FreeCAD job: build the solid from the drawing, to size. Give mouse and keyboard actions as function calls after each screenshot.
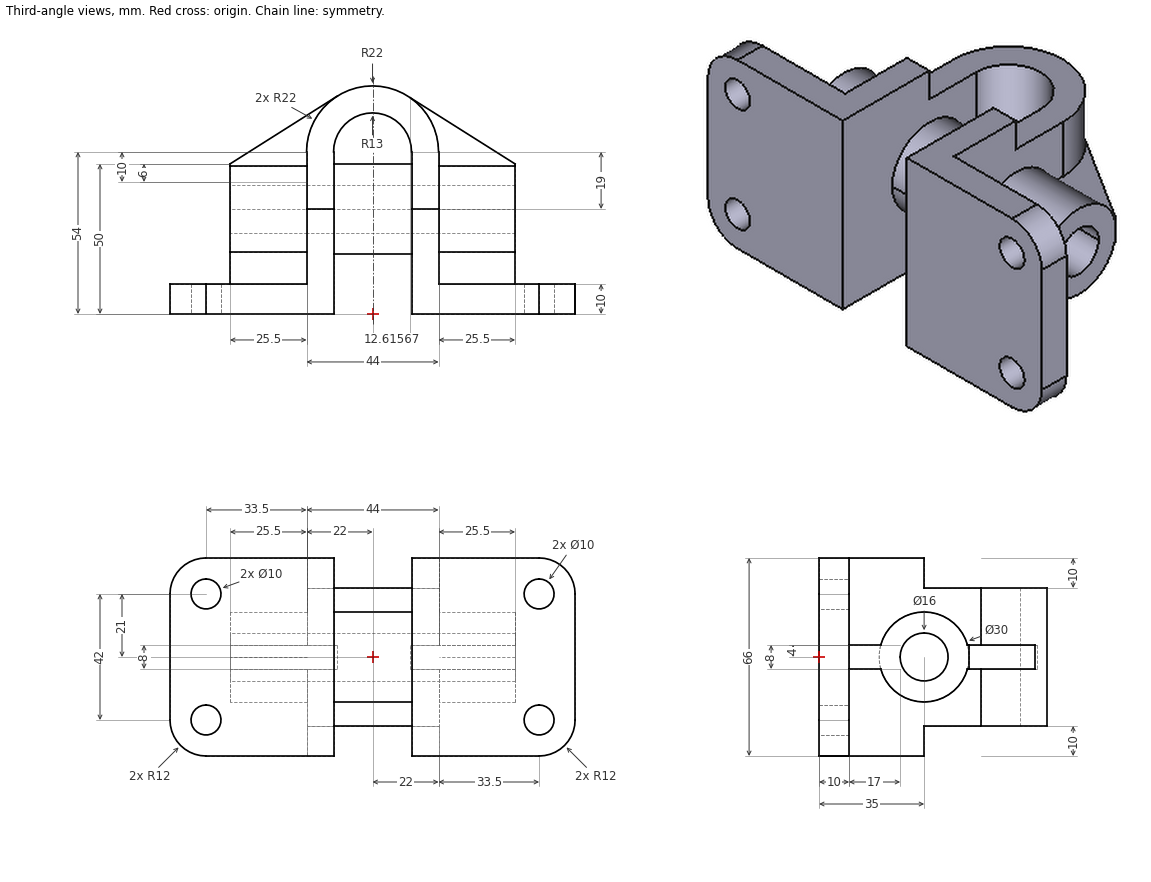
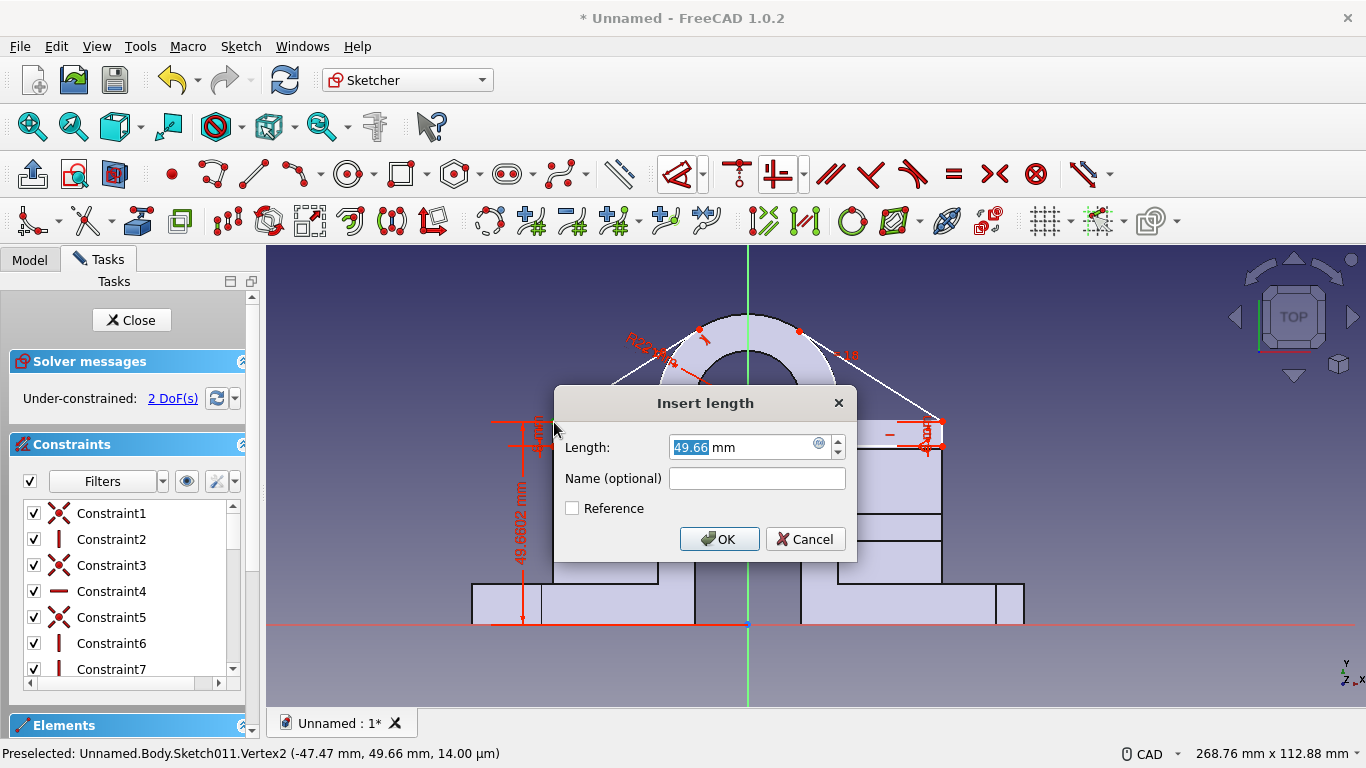
text(50)
key(Return)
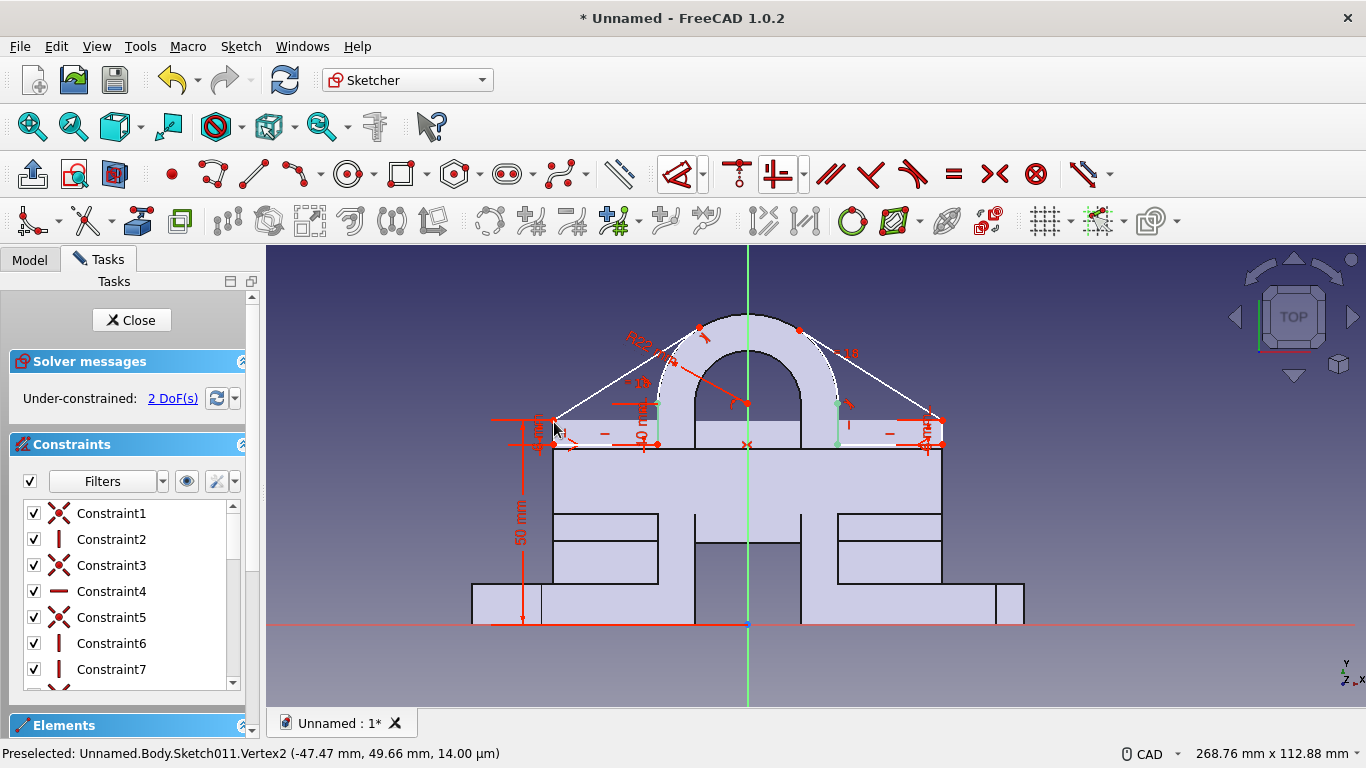
click(585, 445)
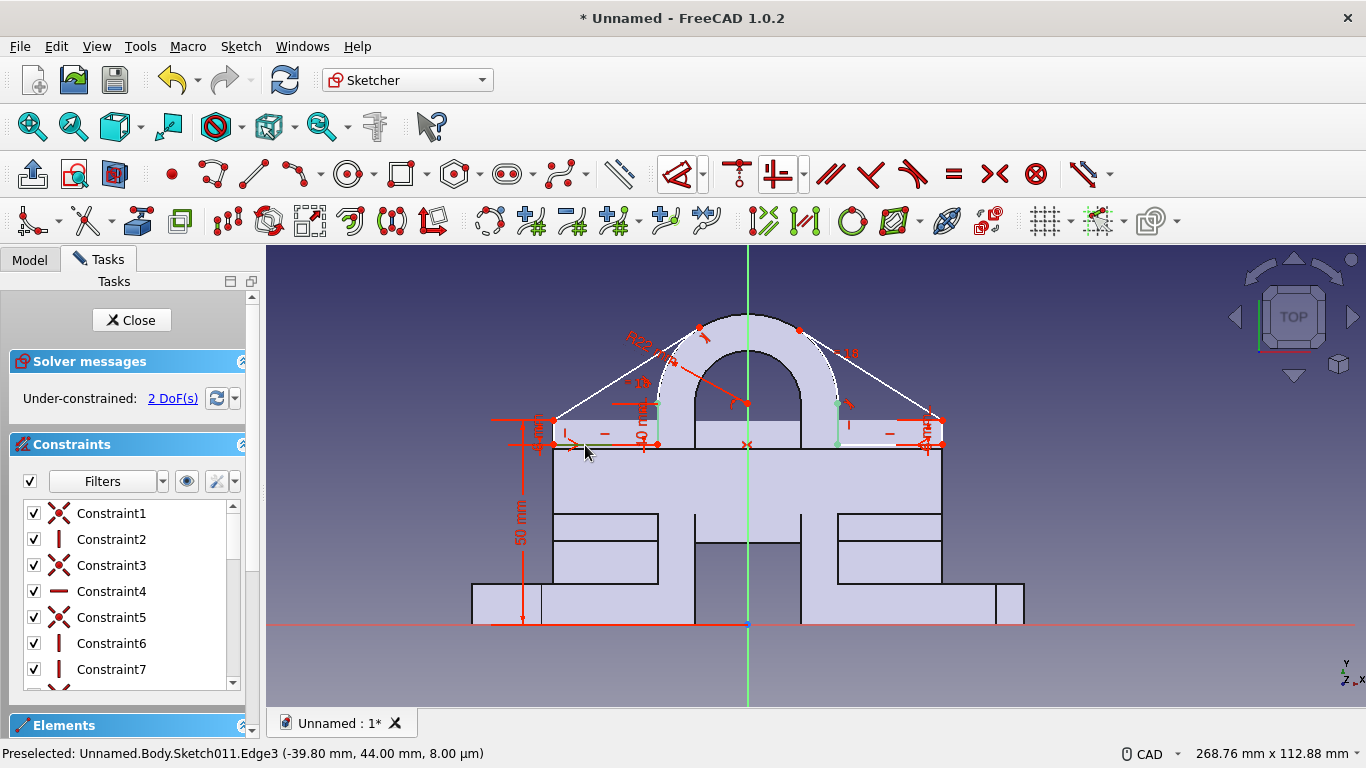
key(l)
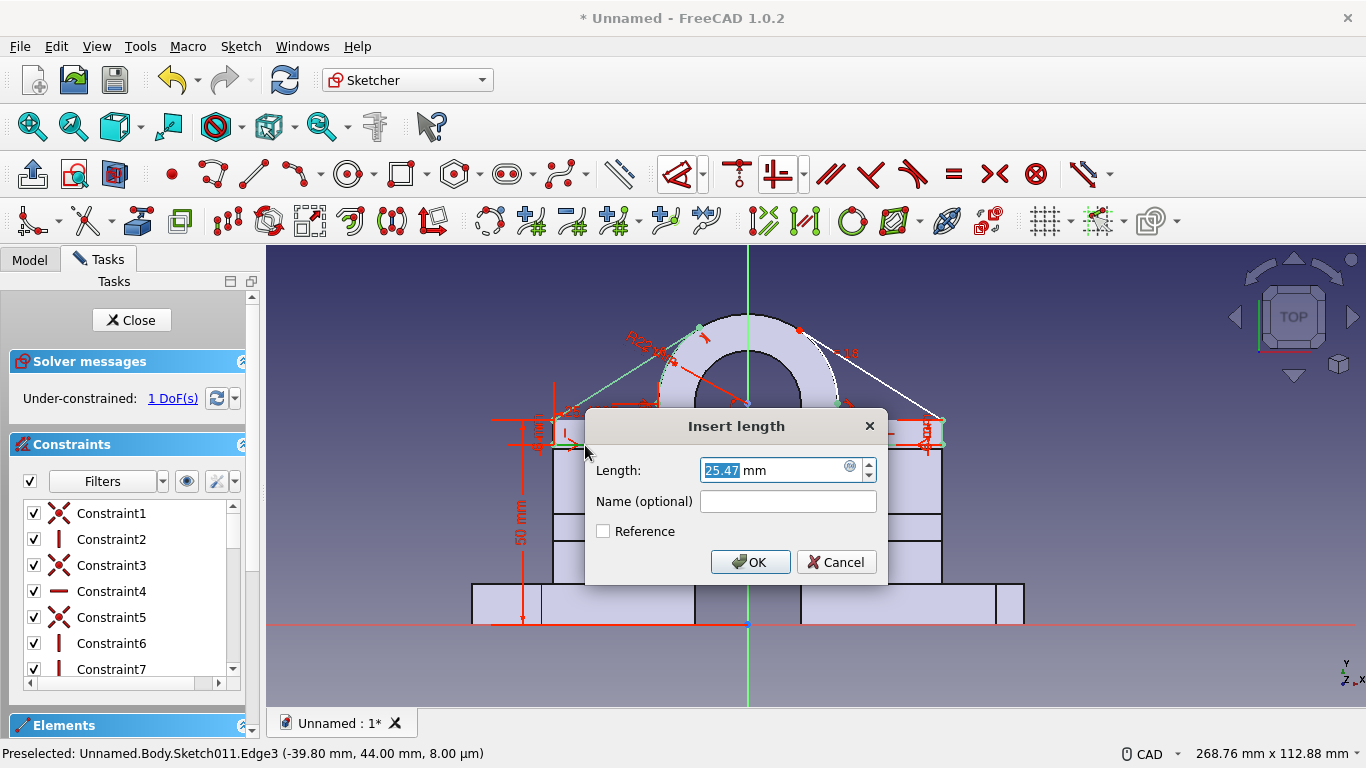
text(25.5)
key(Return)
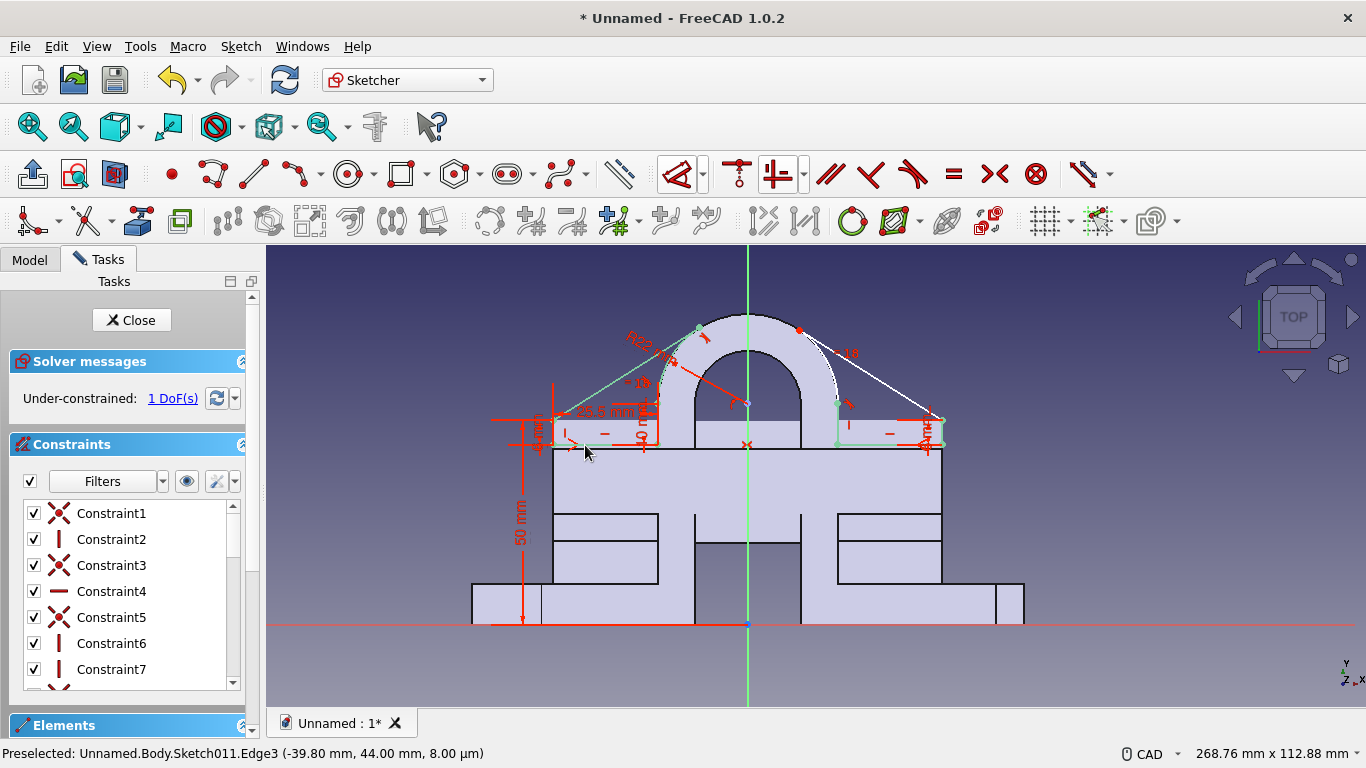
click(799, 330)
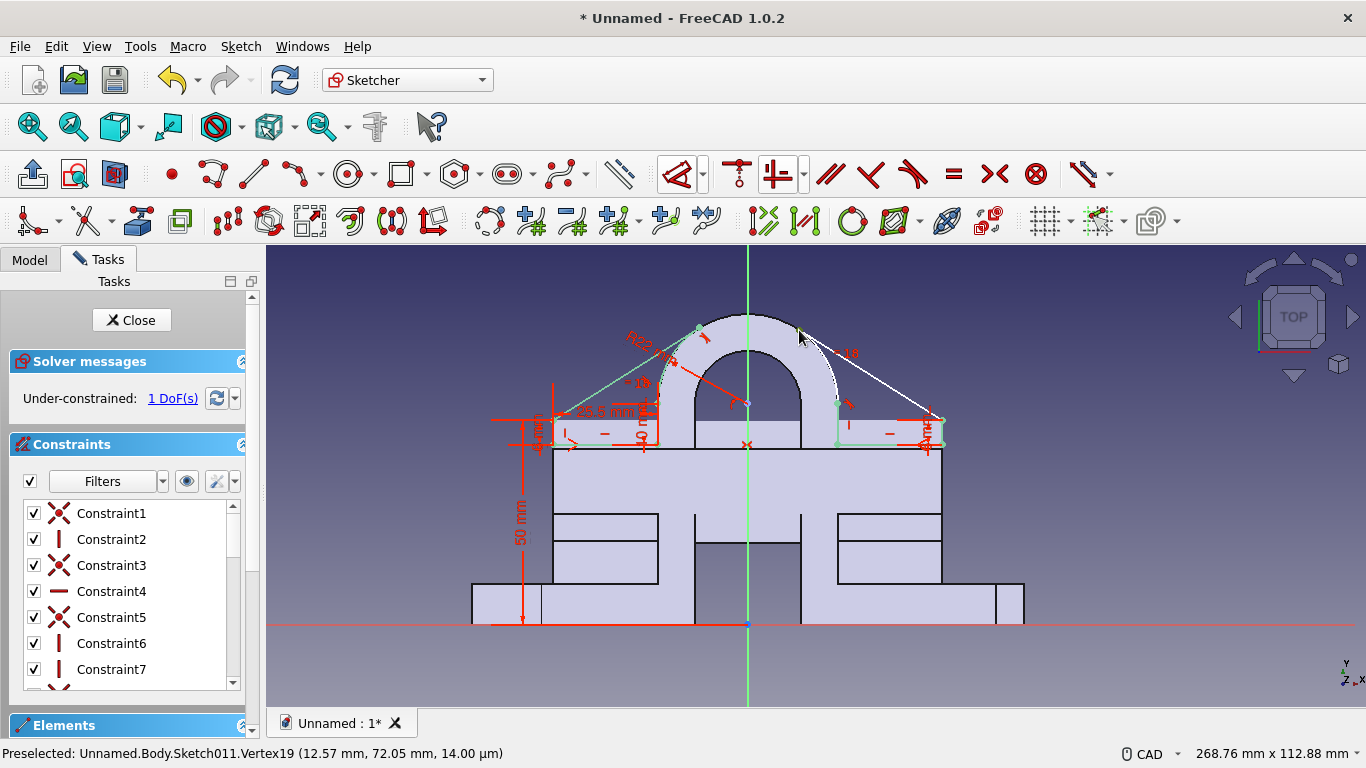
click(702, 174)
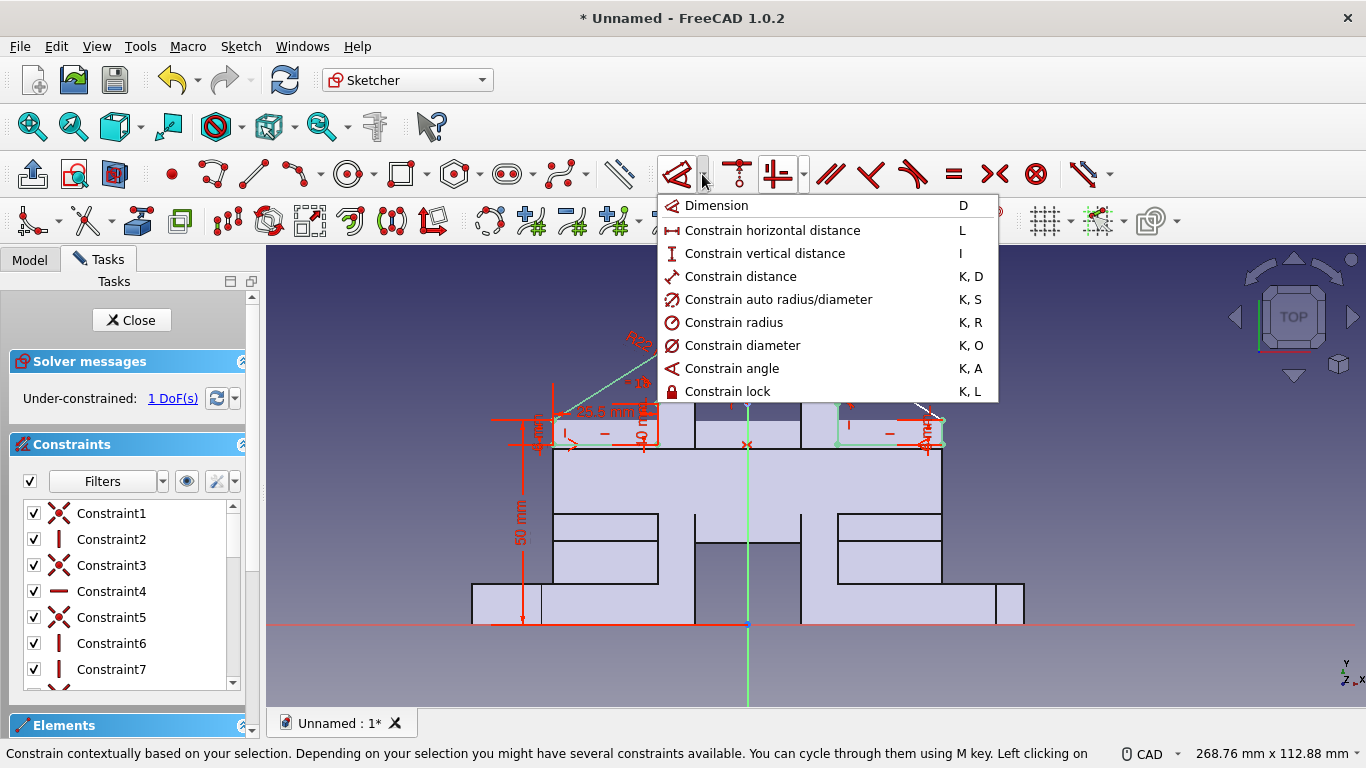
click(828, 230)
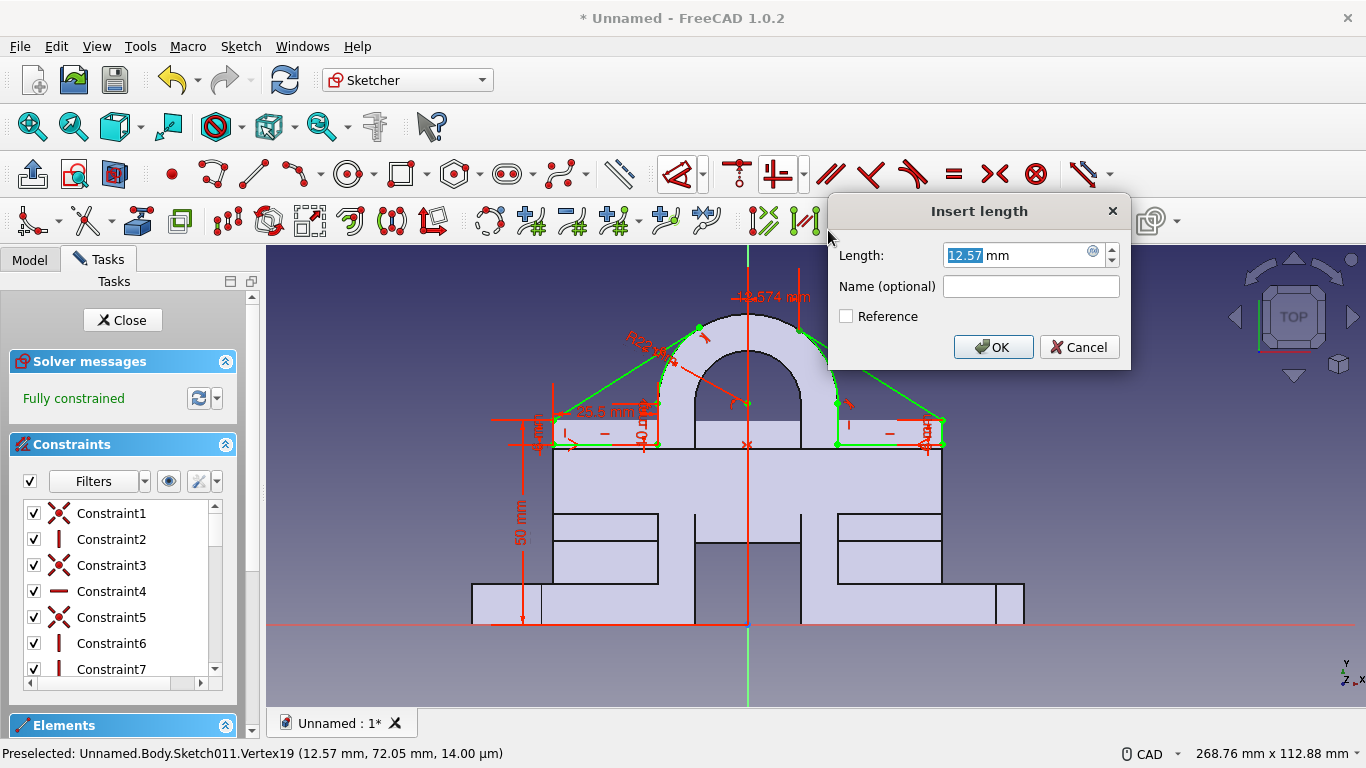
text(12.61567)
key(Return)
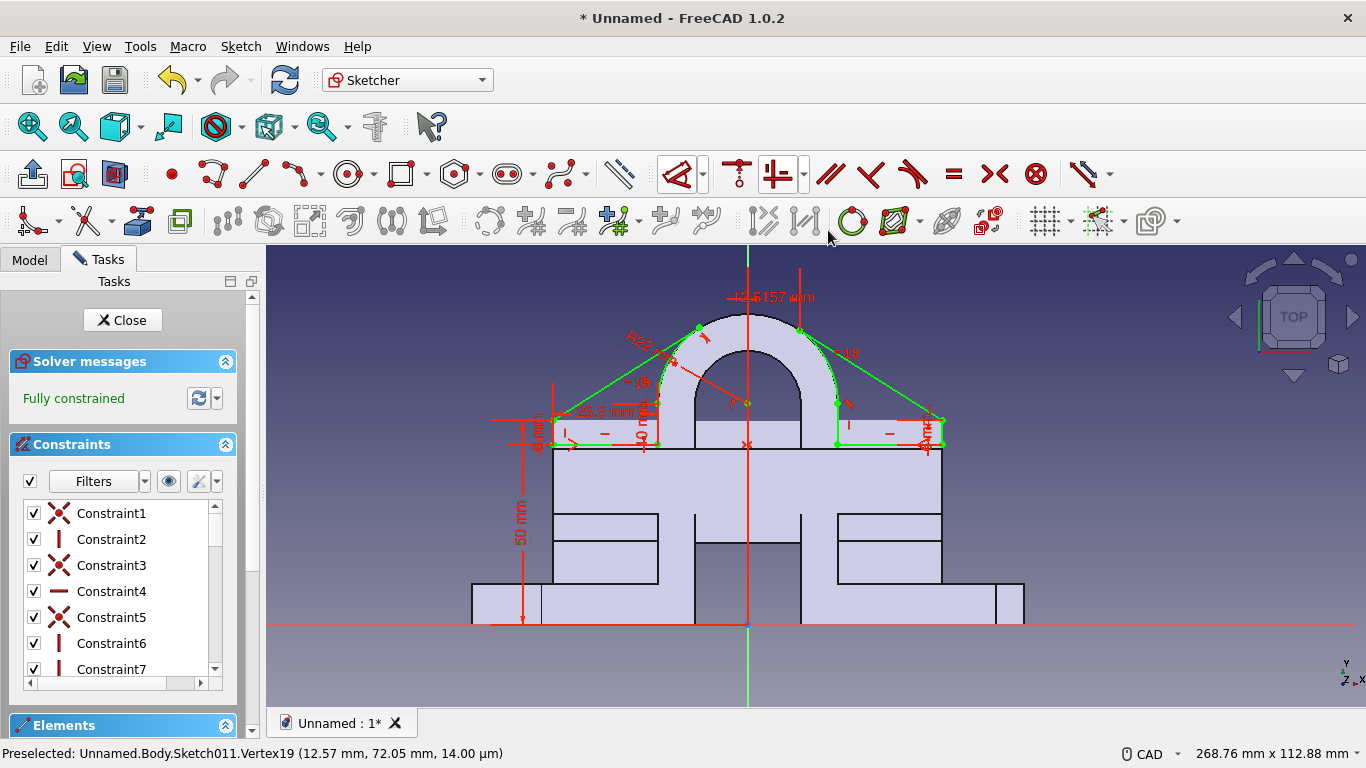
click(123, 320)